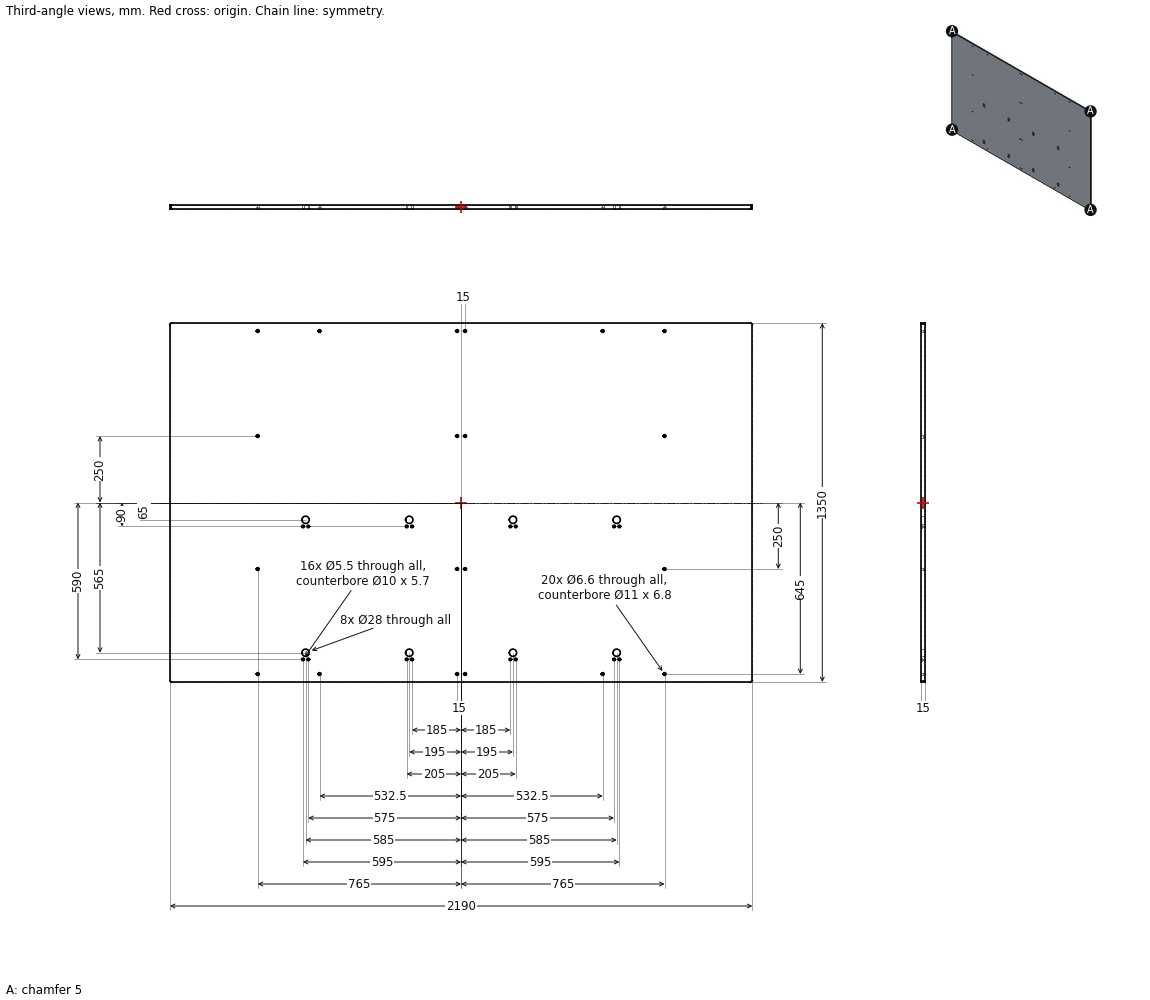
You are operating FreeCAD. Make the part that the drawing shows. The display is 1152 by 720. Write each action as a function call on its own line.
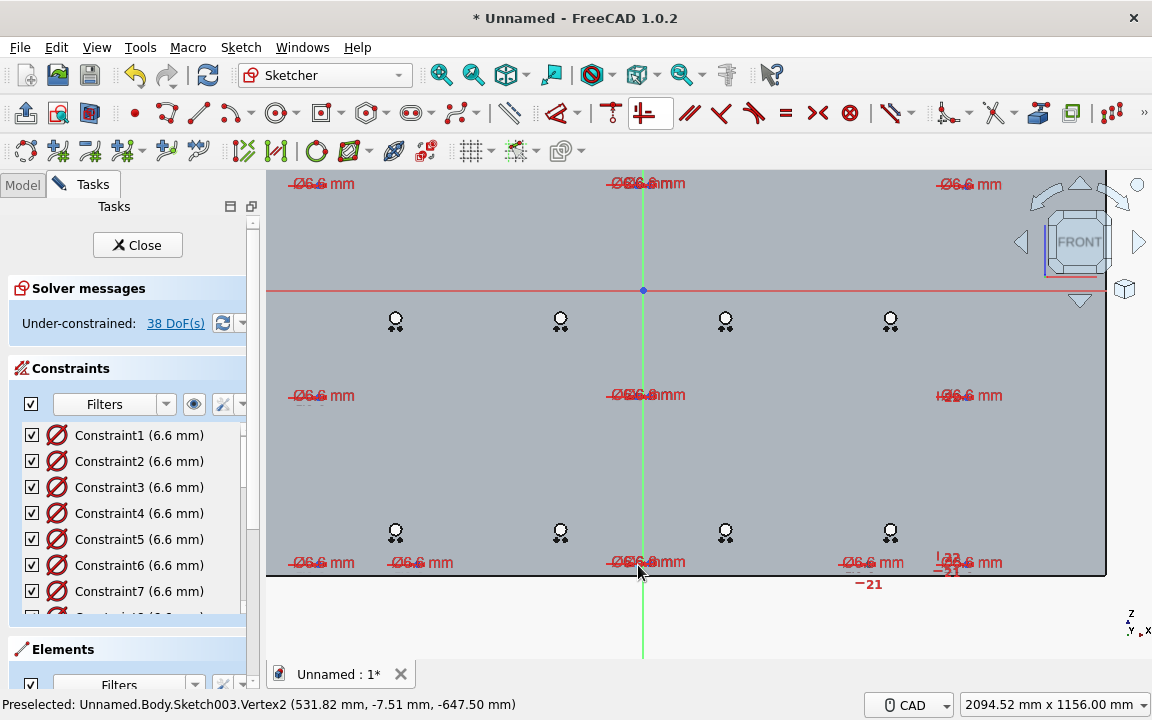
click(637, 564)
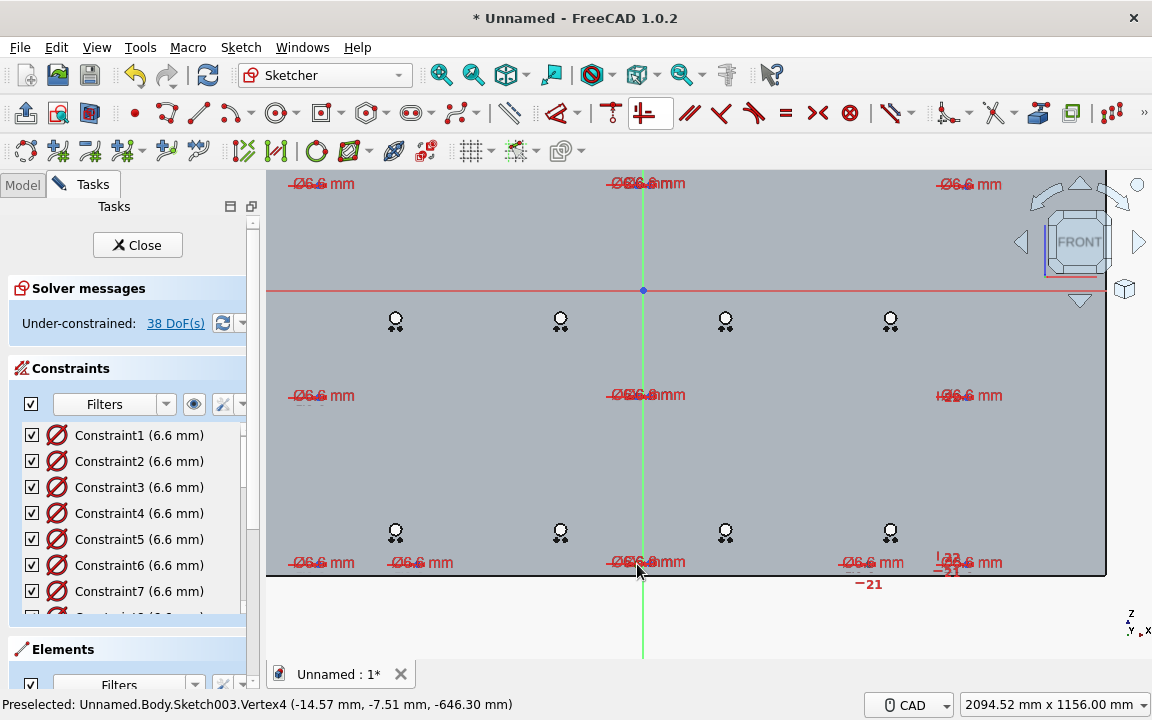
key(h)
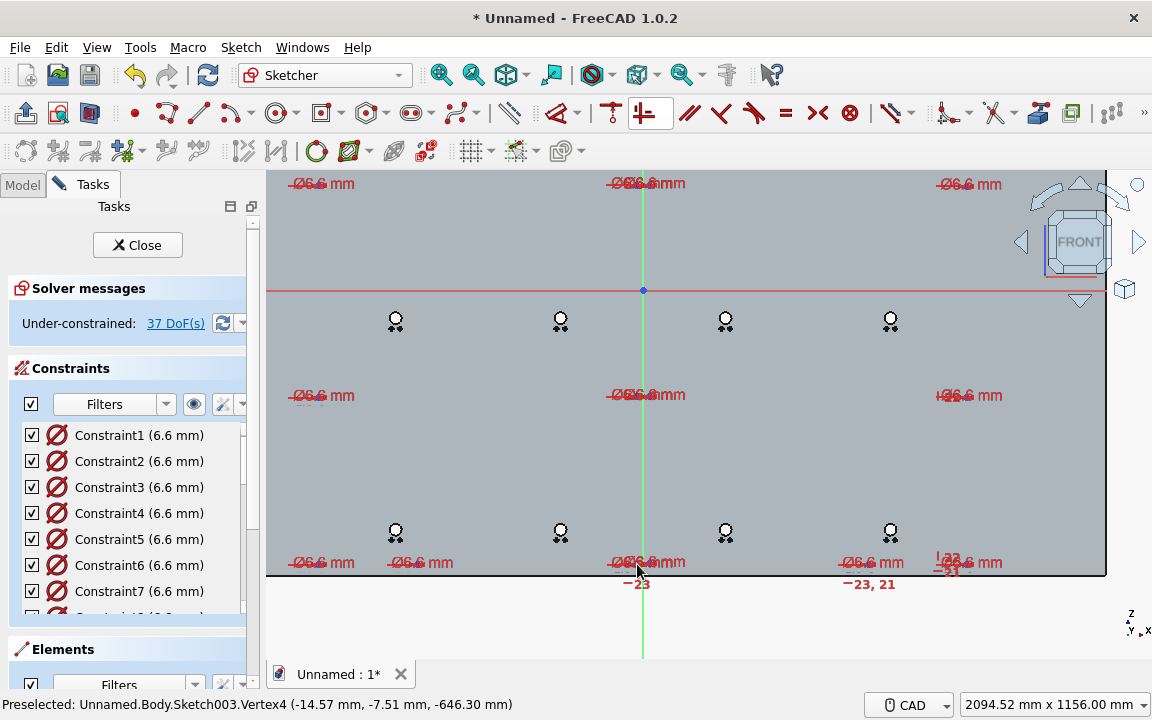
click(637, 565)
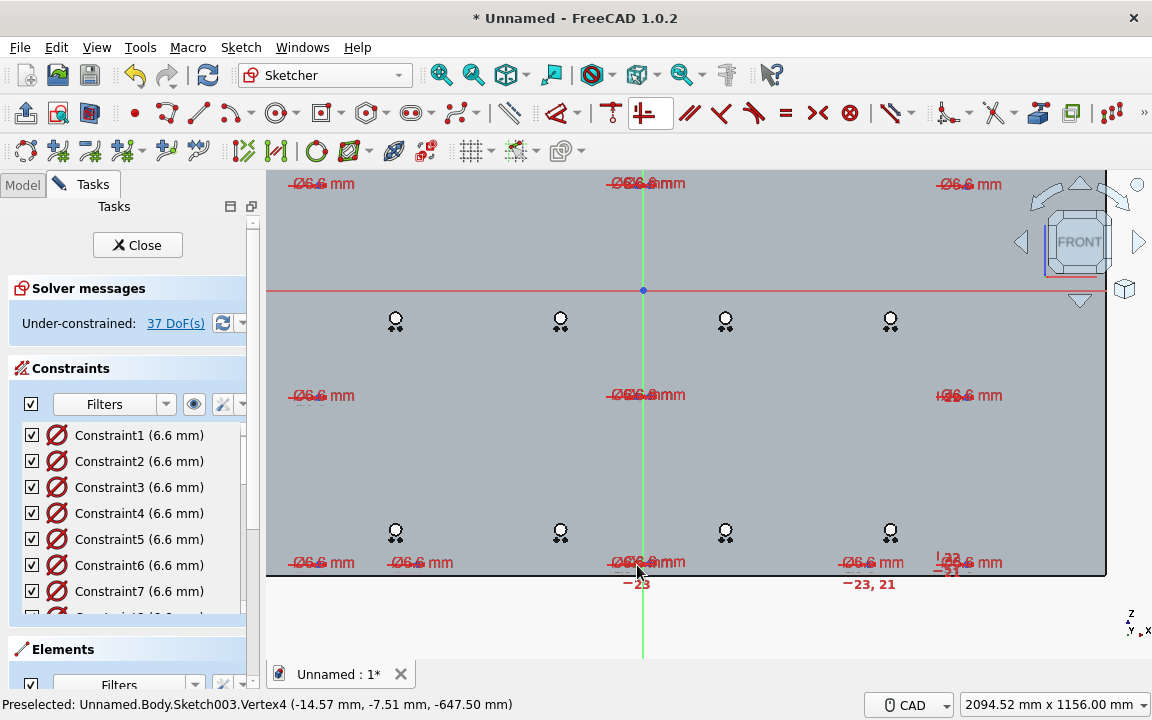
click(637, 397)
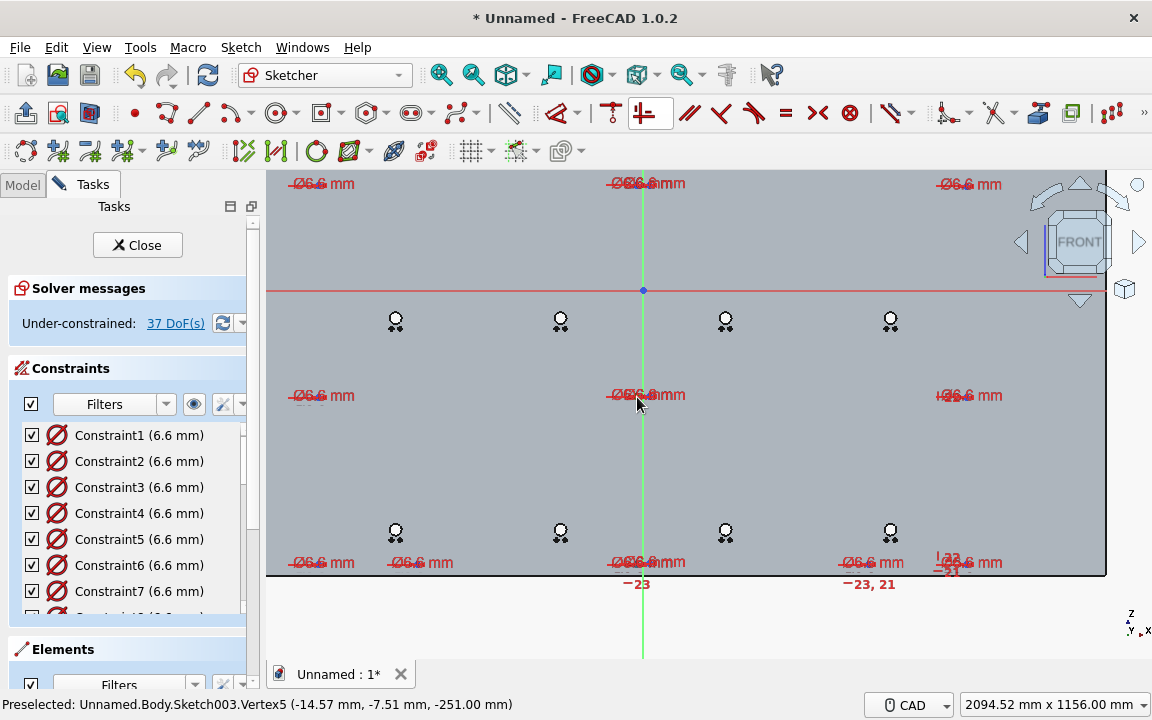
key(v)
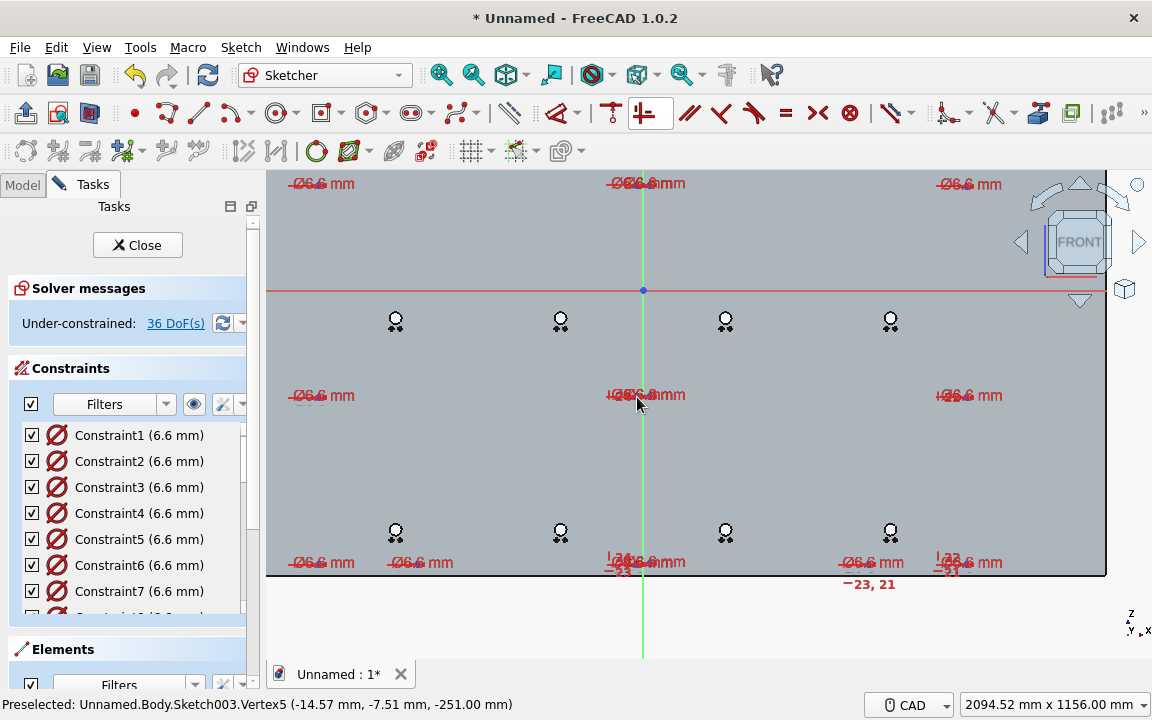
click(967, 397)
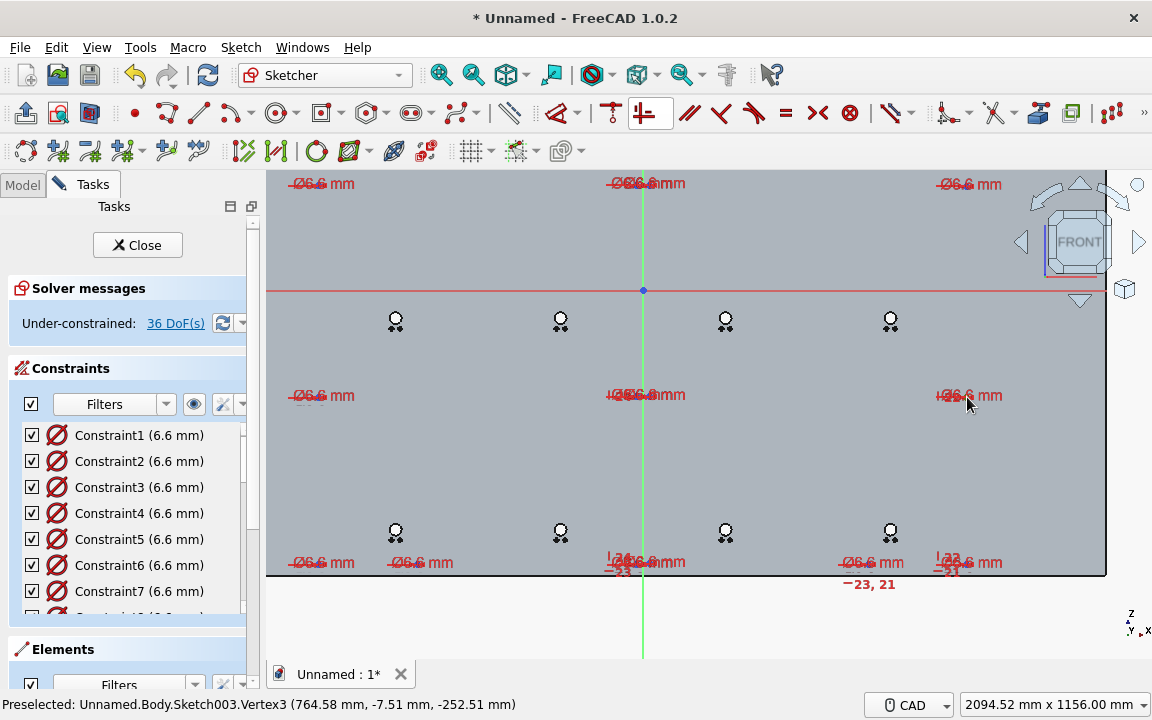
click(637, 397)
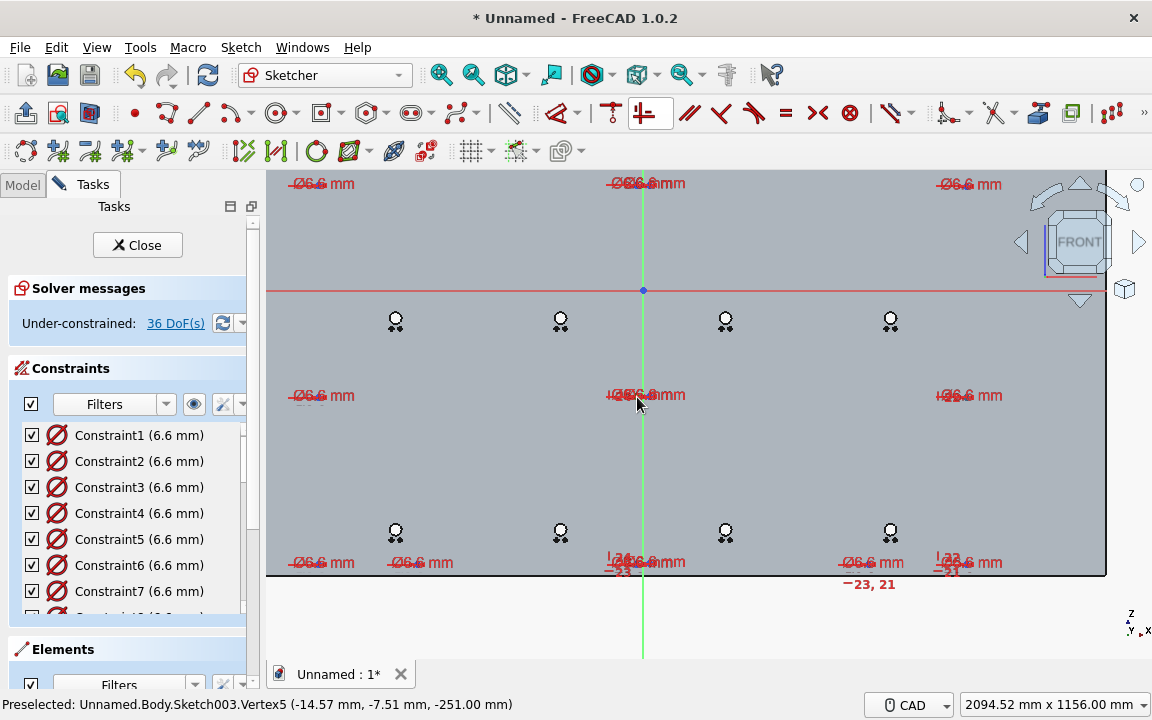
key(h)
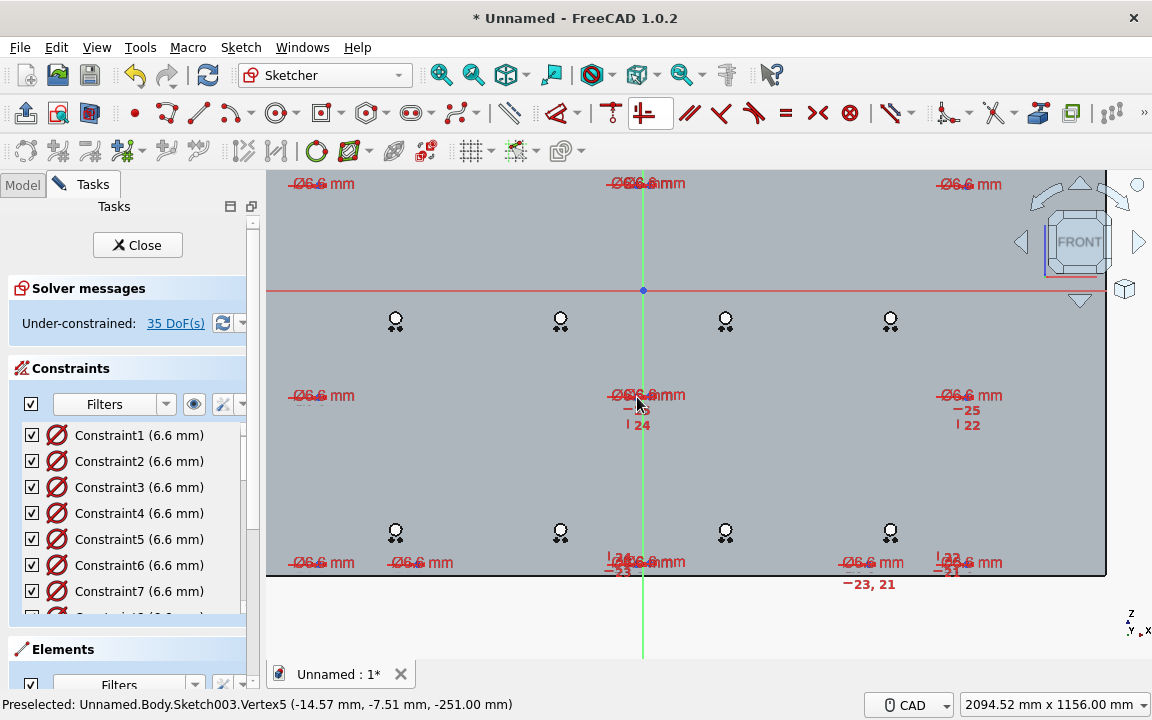
click(637, 397)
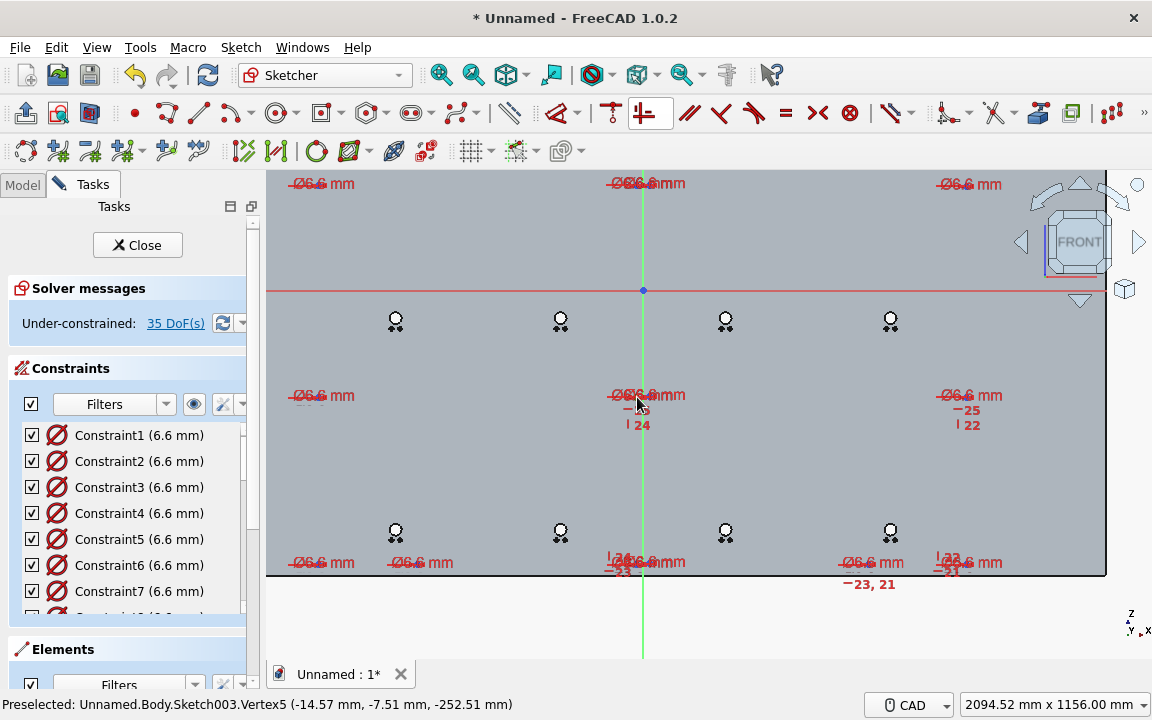
click(319, 398)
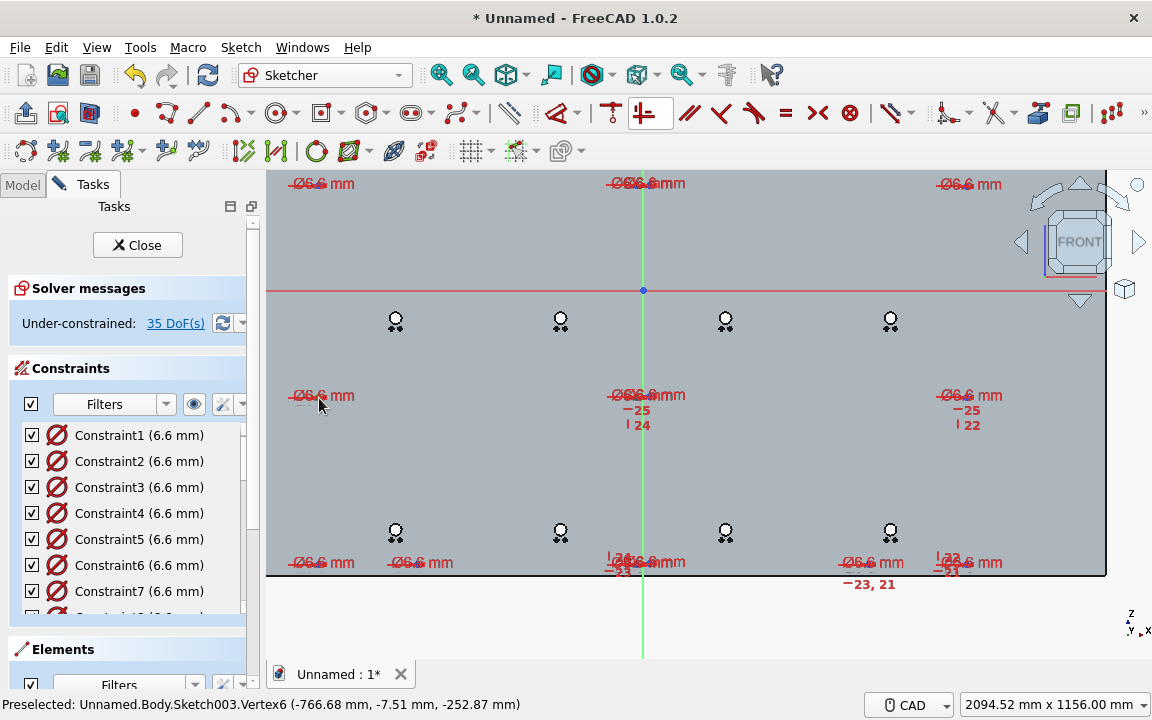
key(h)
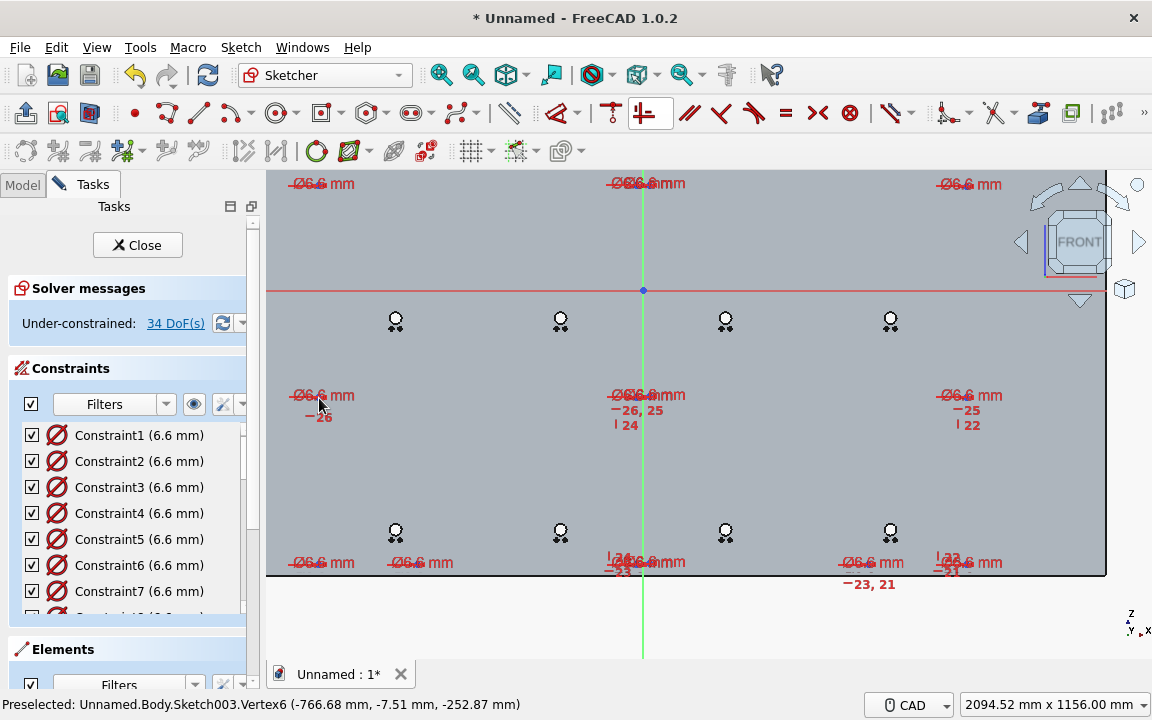
click(637, 565)